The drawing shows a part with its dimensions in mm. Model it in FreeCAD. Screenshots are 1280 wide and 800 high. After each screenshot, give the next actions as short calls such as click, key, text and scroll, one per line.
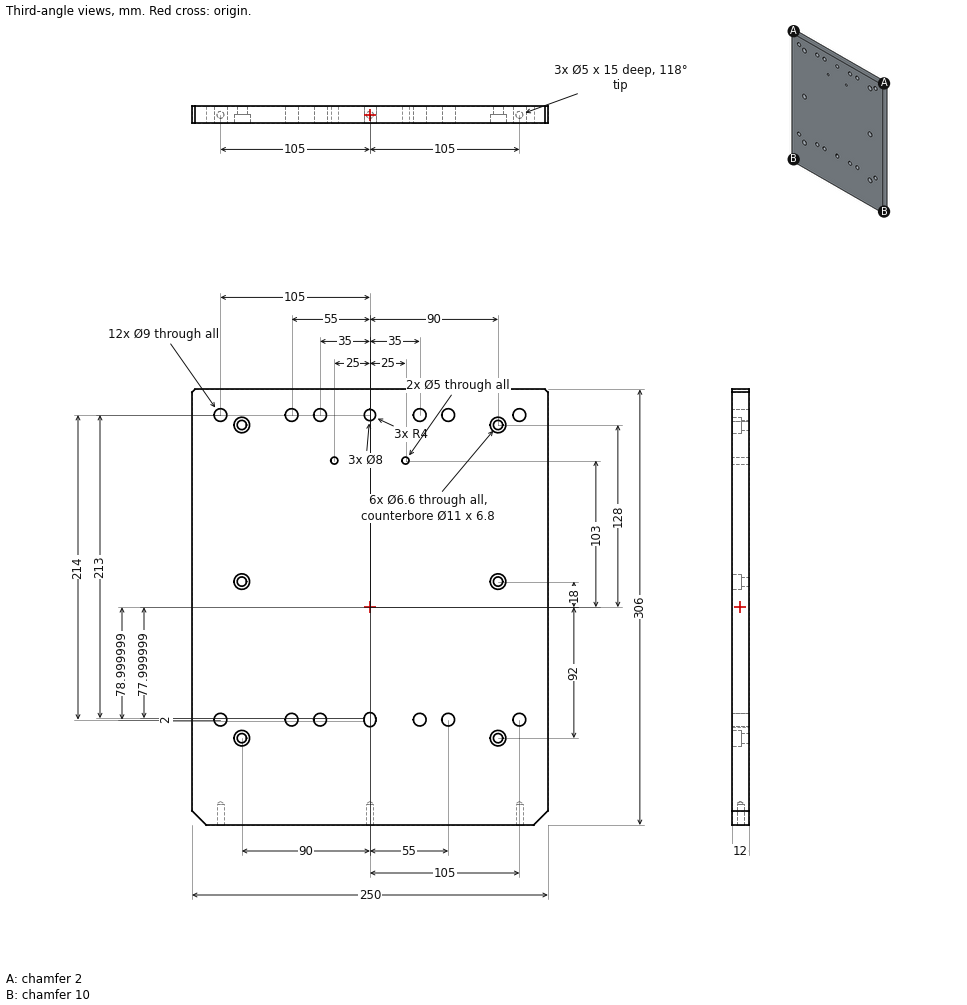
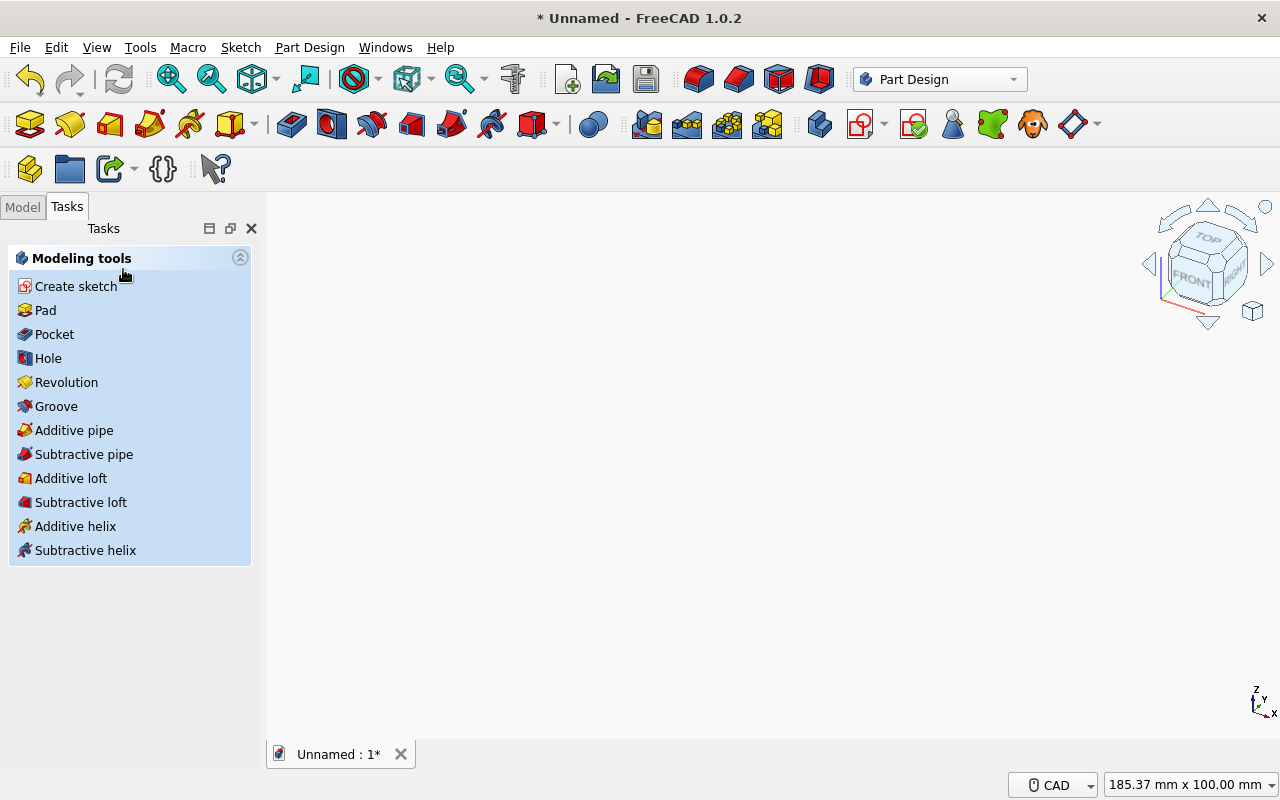
click(30, 124)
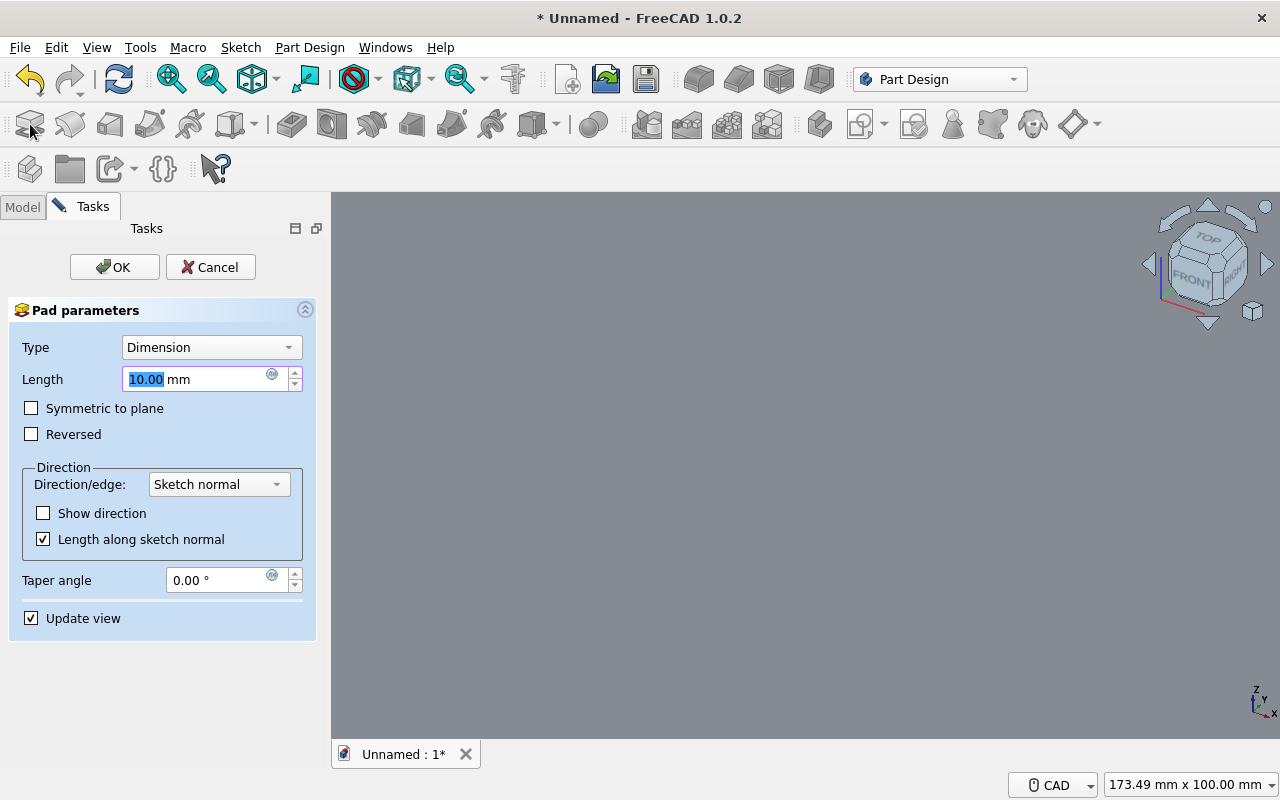
text(12)
key(Tab)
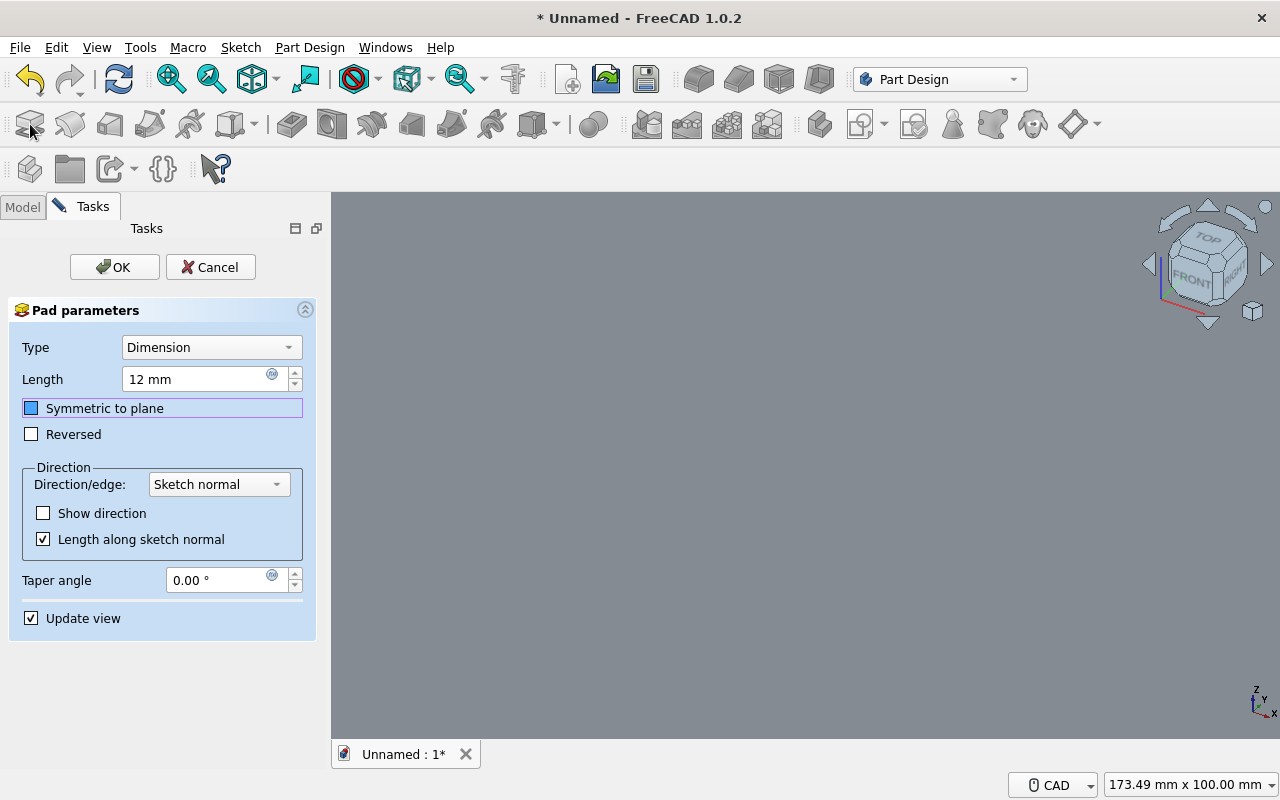
click(30, 408)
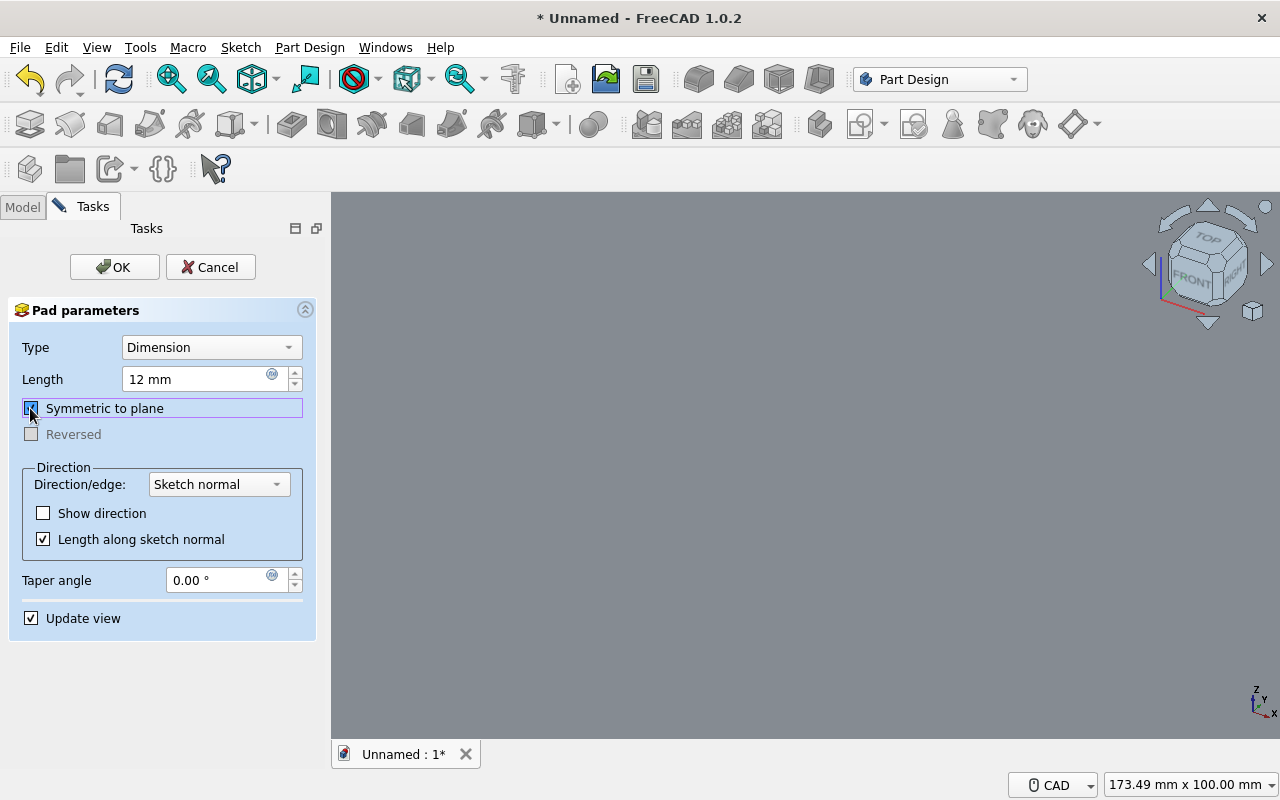
click(115, 267)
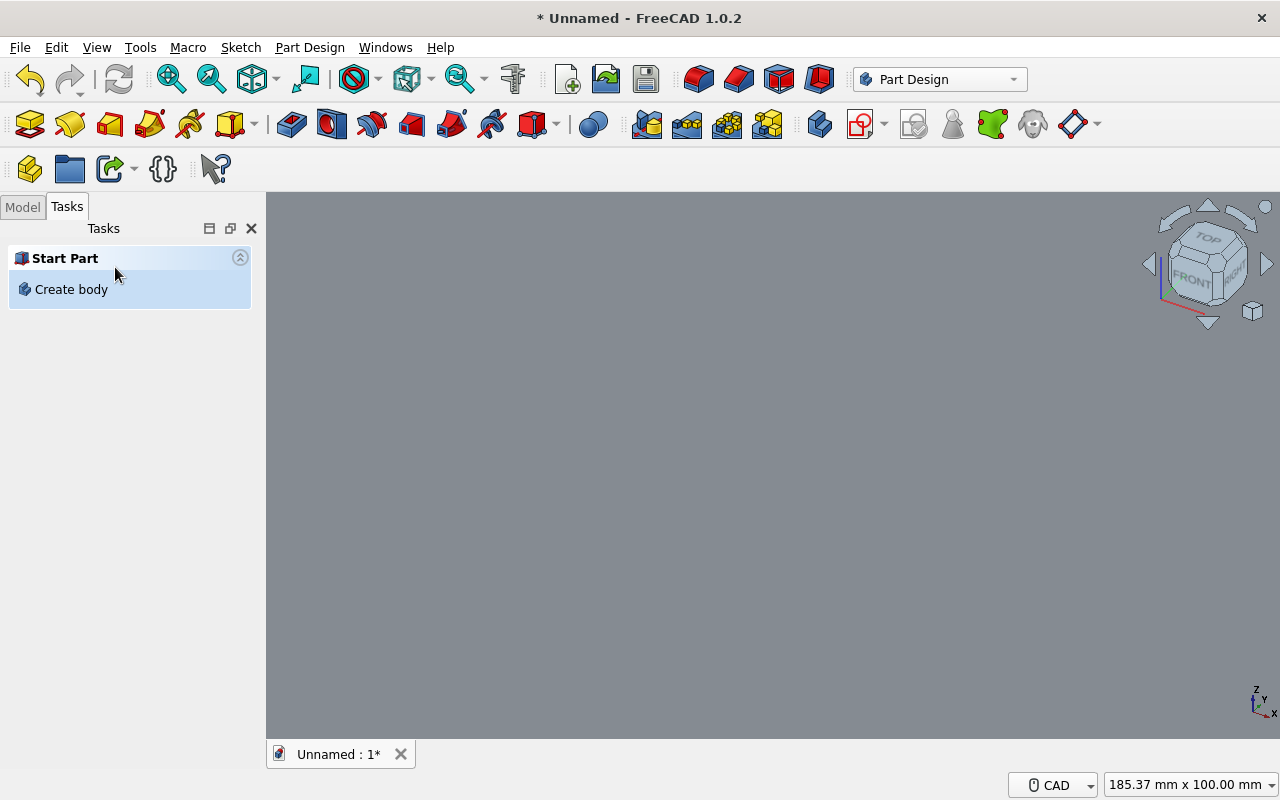
click(172, 80)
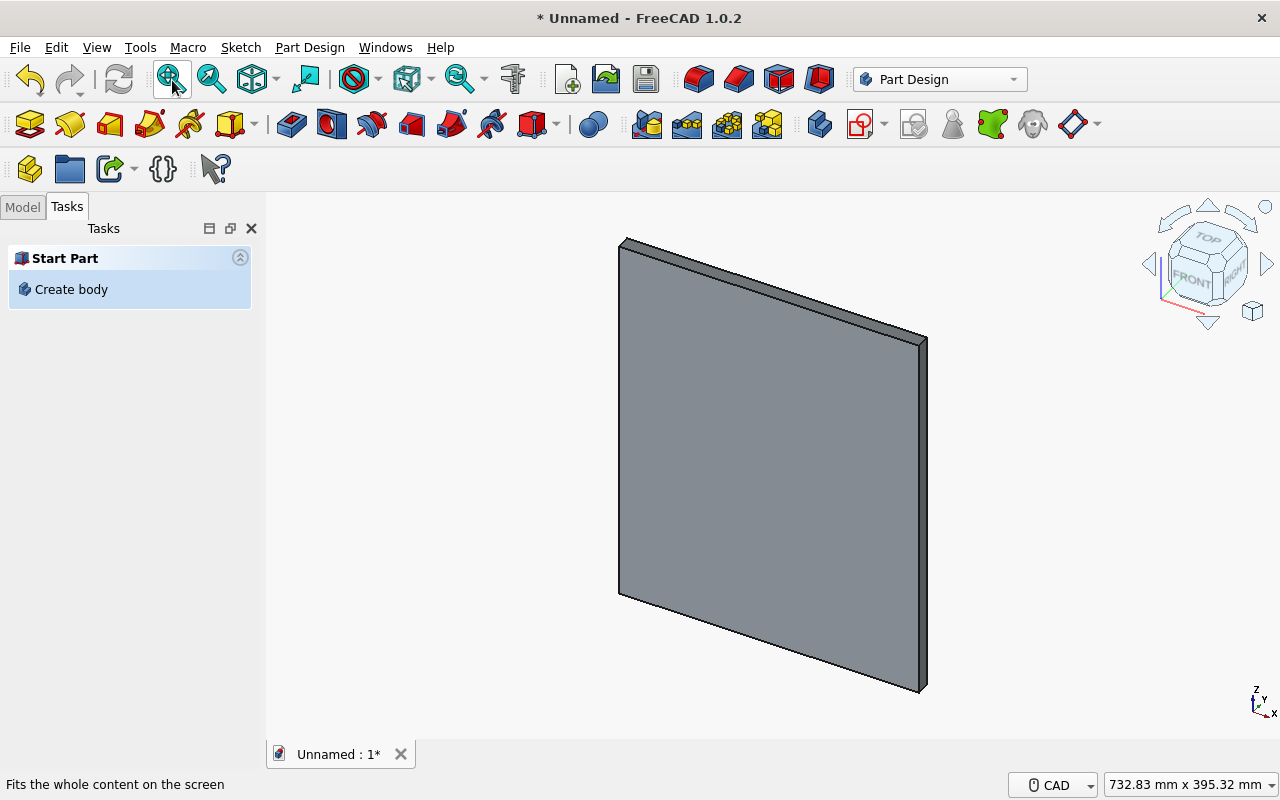
click(924, 340)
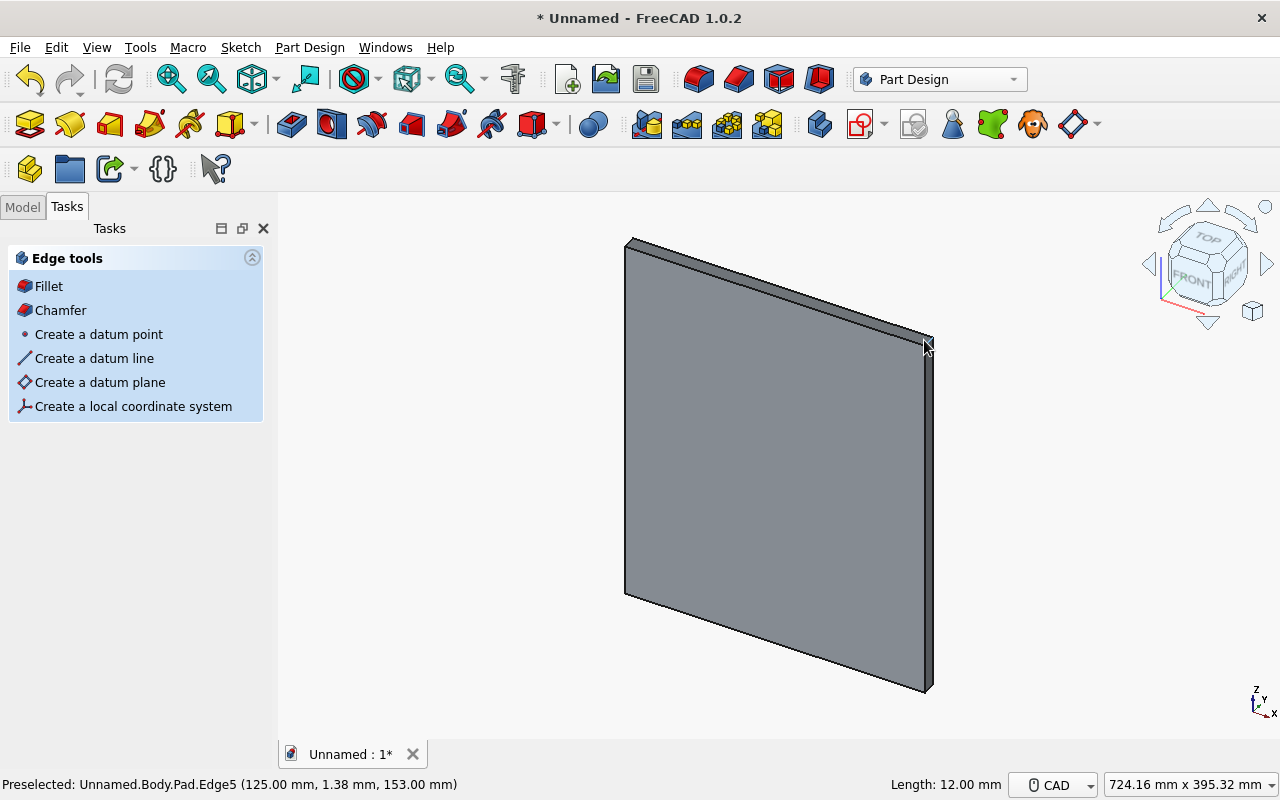
scroll(629, 241, up, 5)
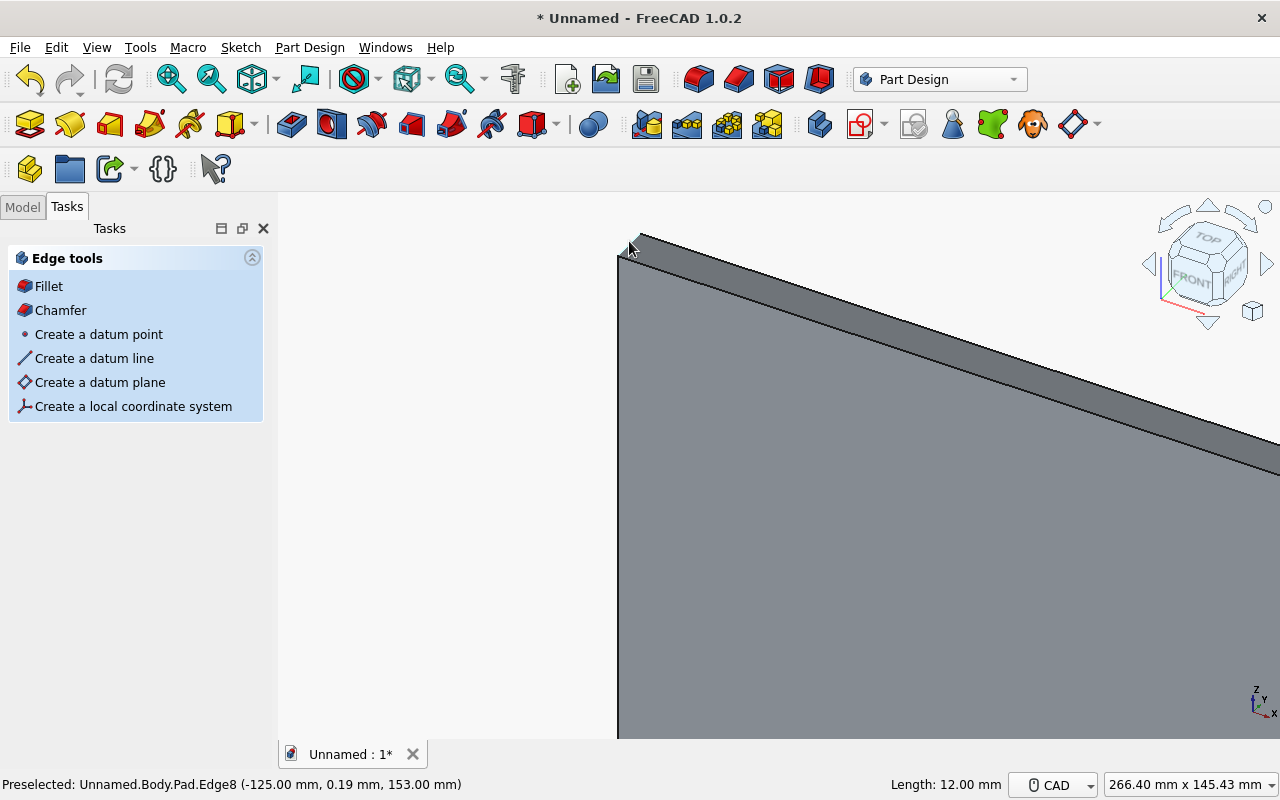
click(172, 80)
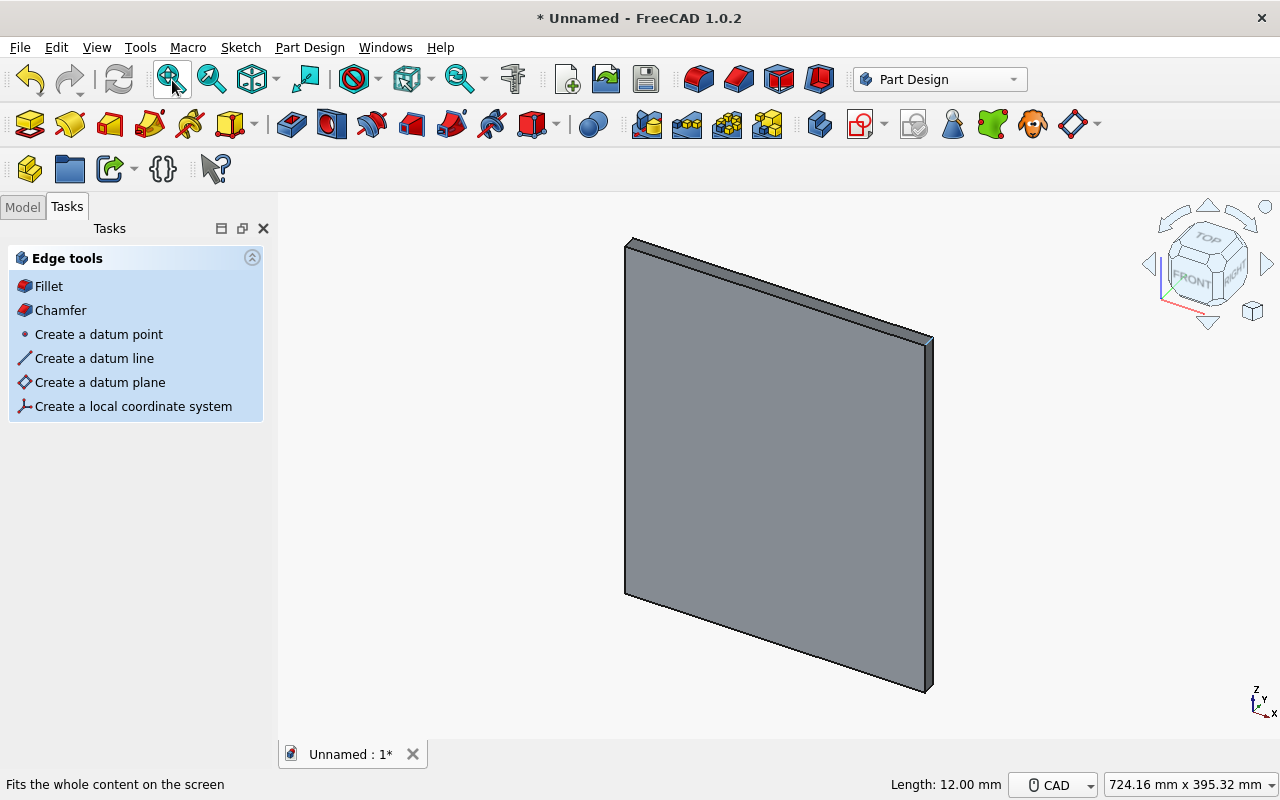
key(0)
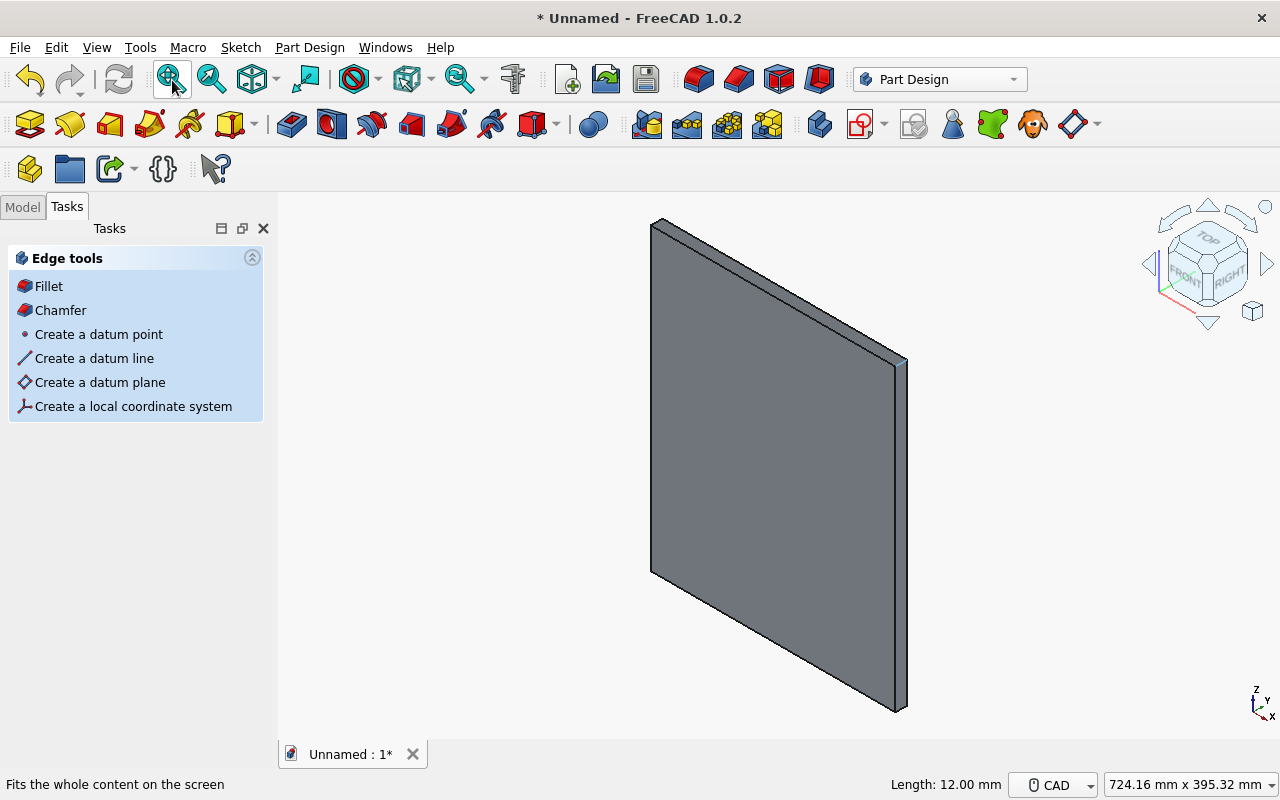
scroll(657, 221, up, 5)